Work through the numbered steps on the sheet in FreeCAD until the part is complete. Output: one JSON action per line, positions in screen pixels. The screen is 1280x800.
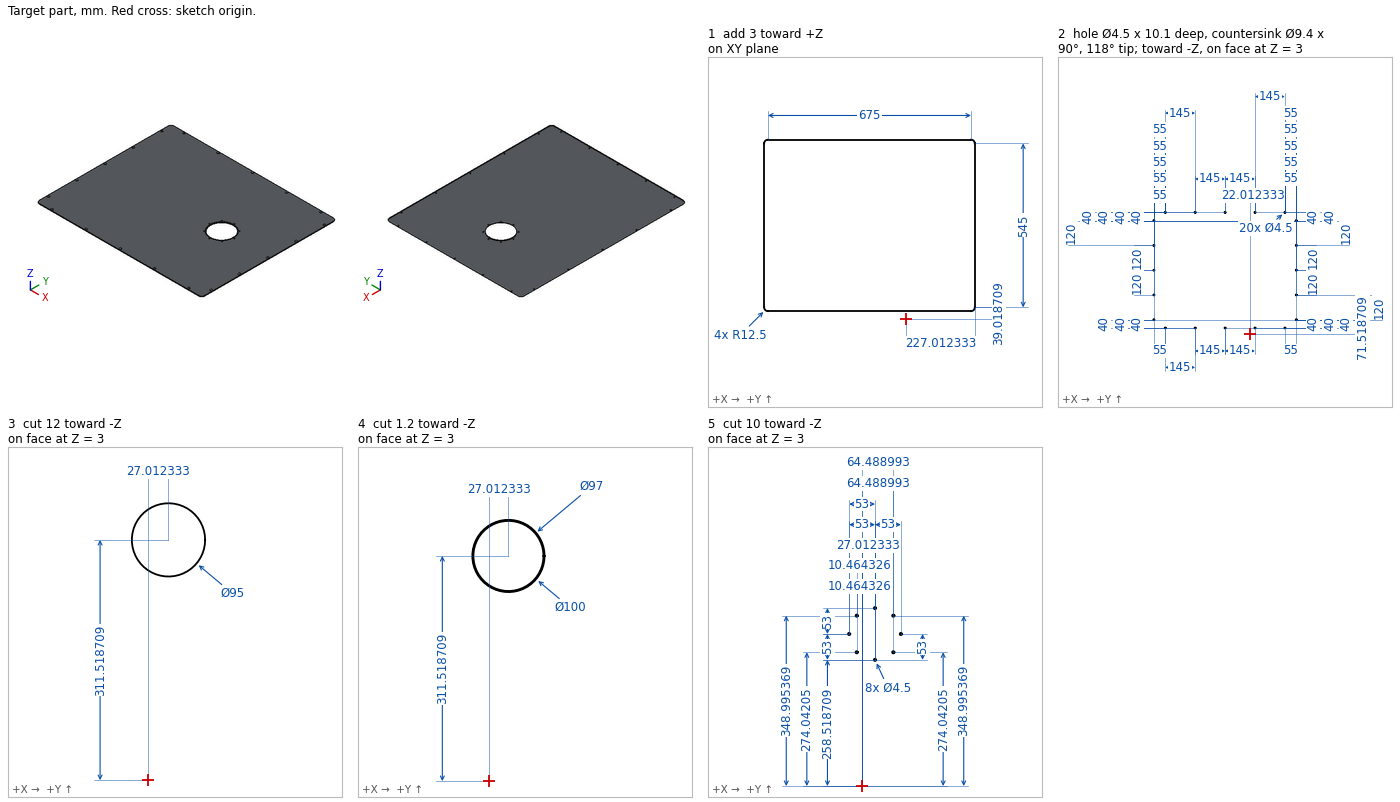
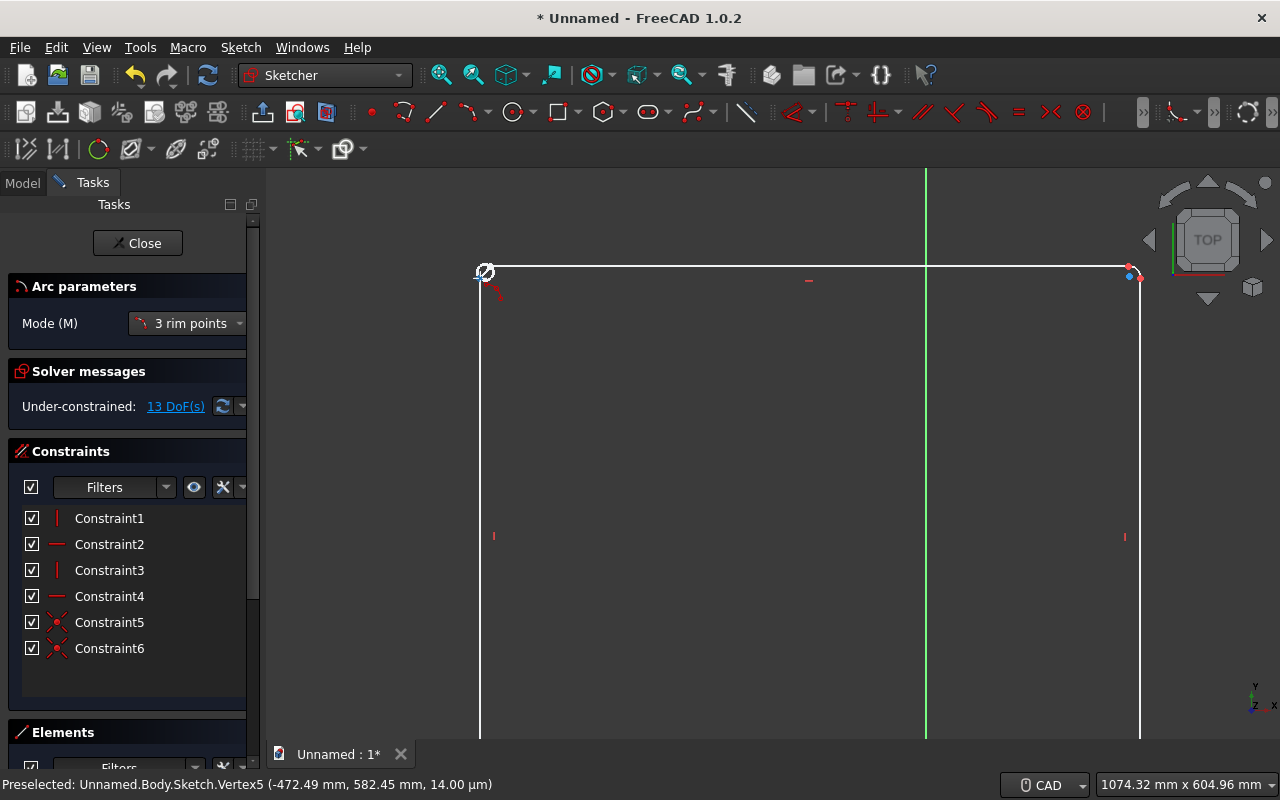
{"action": "scroll", "coordinate": [483, 269], "scroll_direction": "up", "scroll_amount": 8}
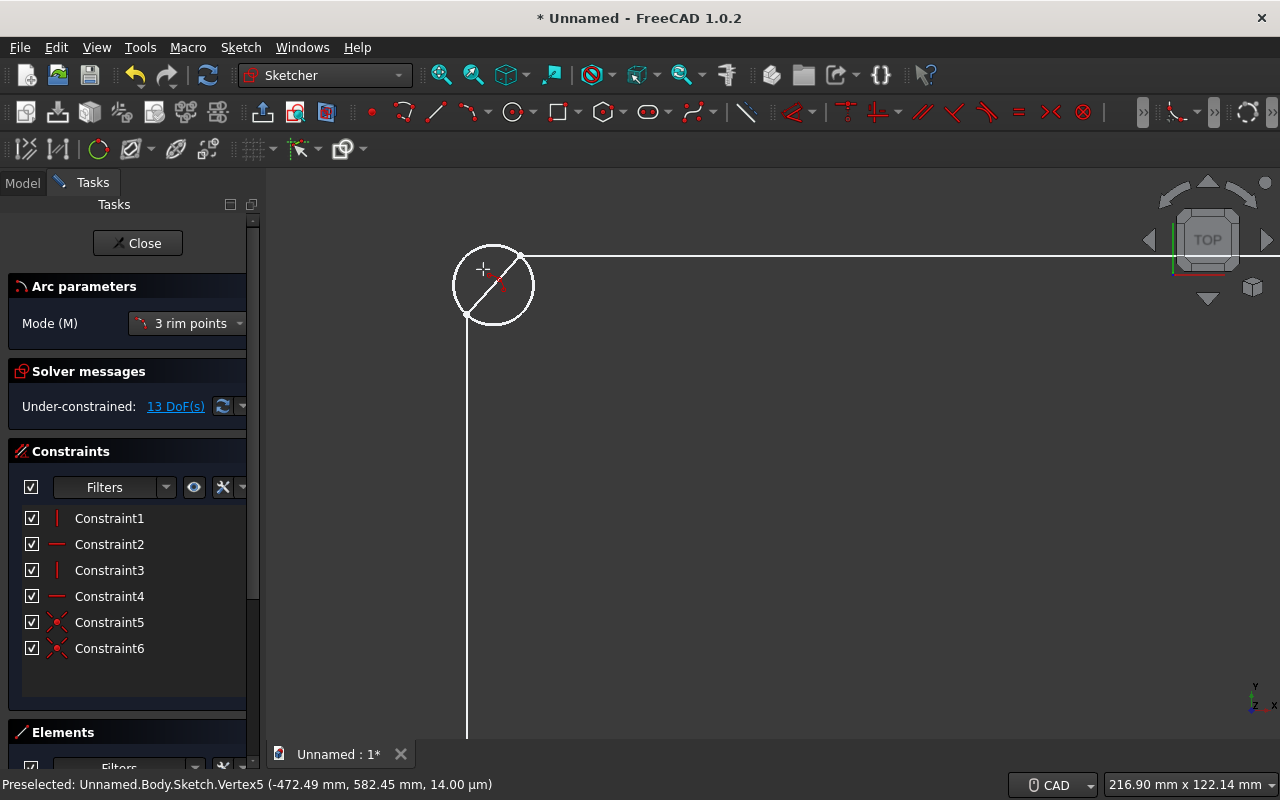
{"action": "left_click", "coordinate": [481, 266]}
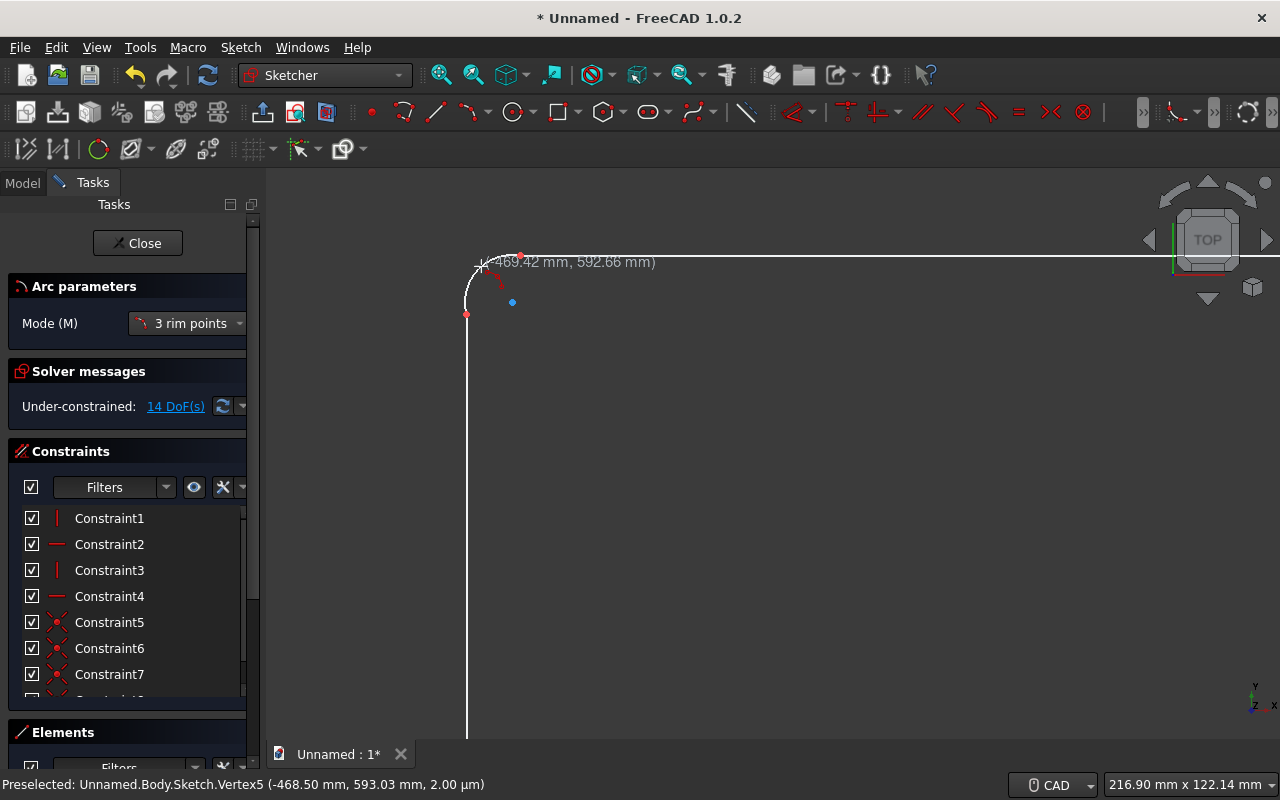
{"action": "scroll", "coordinate": [486, 267], "scroll_direction": "down", "scroll_amount": 10}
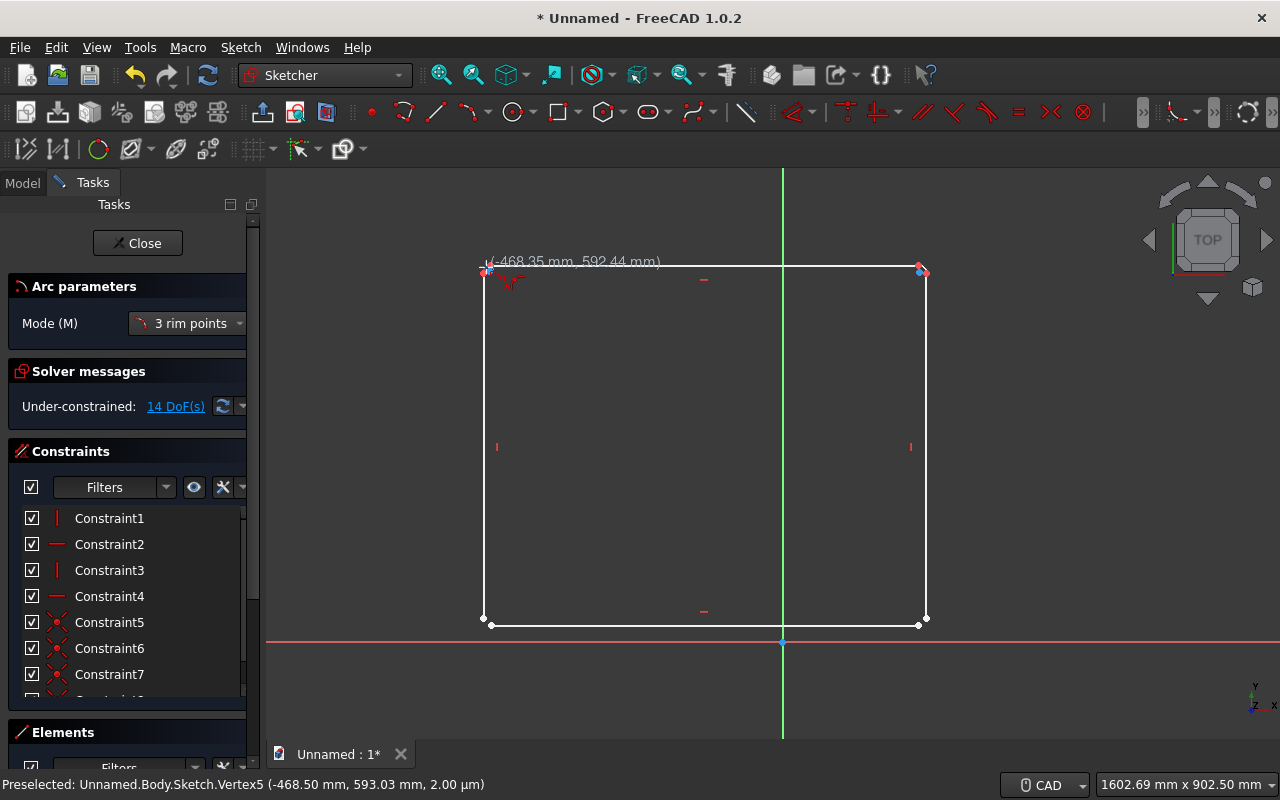
{"action": "scroll", "coordinate": [483, 617], "scroll_direction": "up", "scroll_amount": 2}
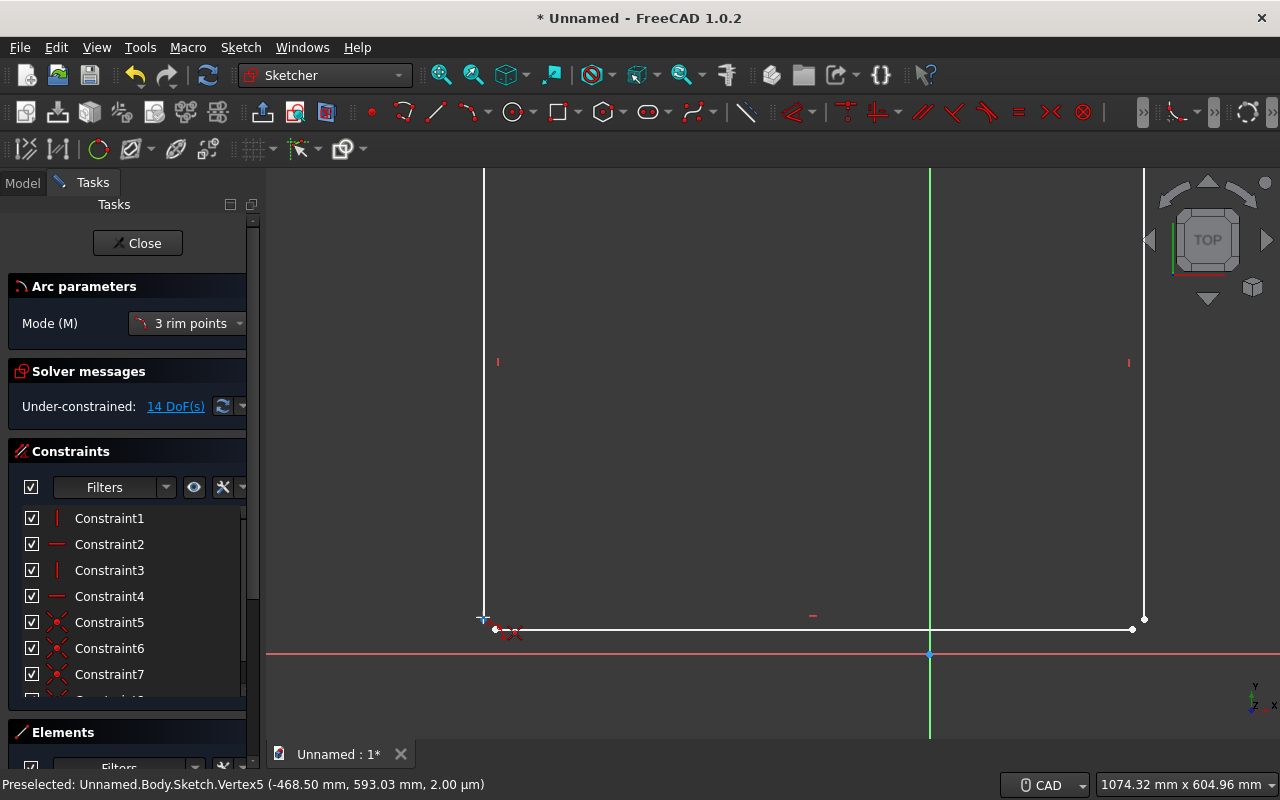
{"action": "left_click", "coordinate": [484, 619]}
{"action": "left_click", "coordinate": [495, 630]}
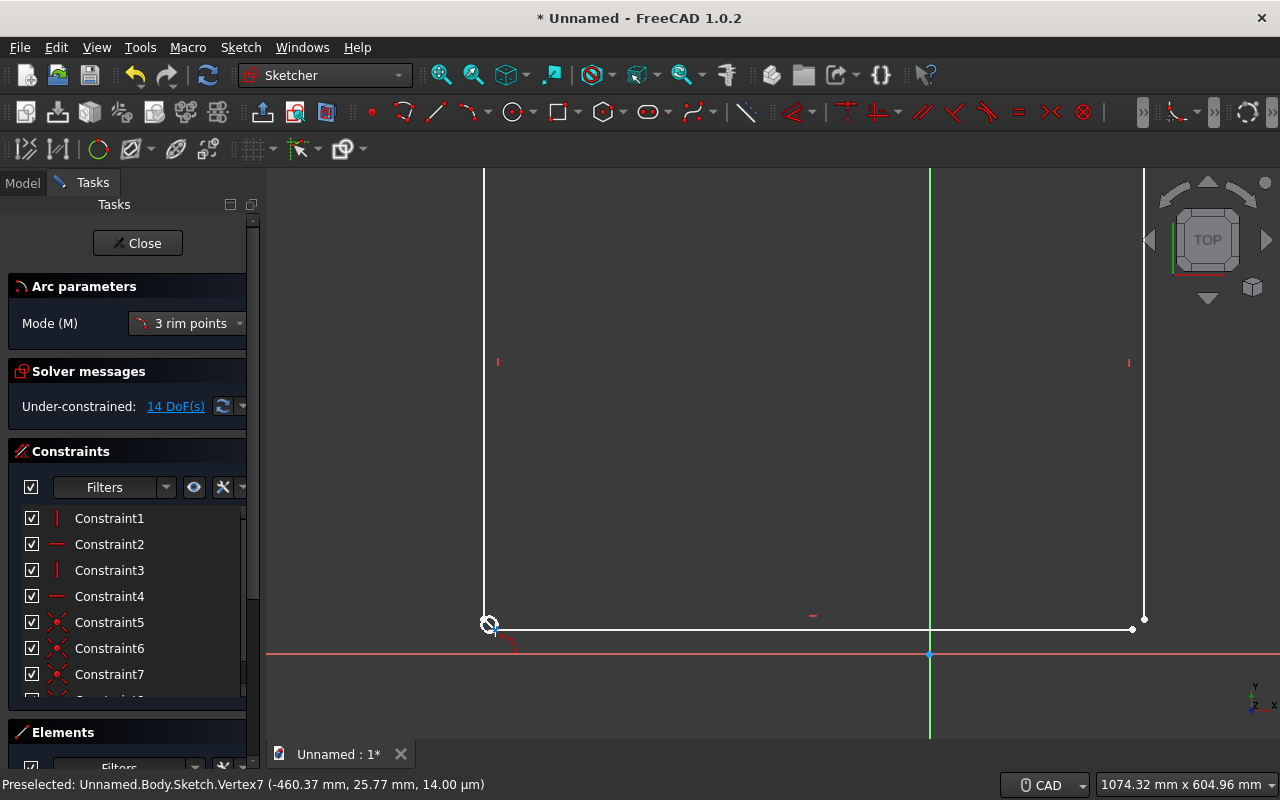
{"action": "scroll", "coordinate": [487, 626], "scroll_direction": "up", "scroll_amount": 8}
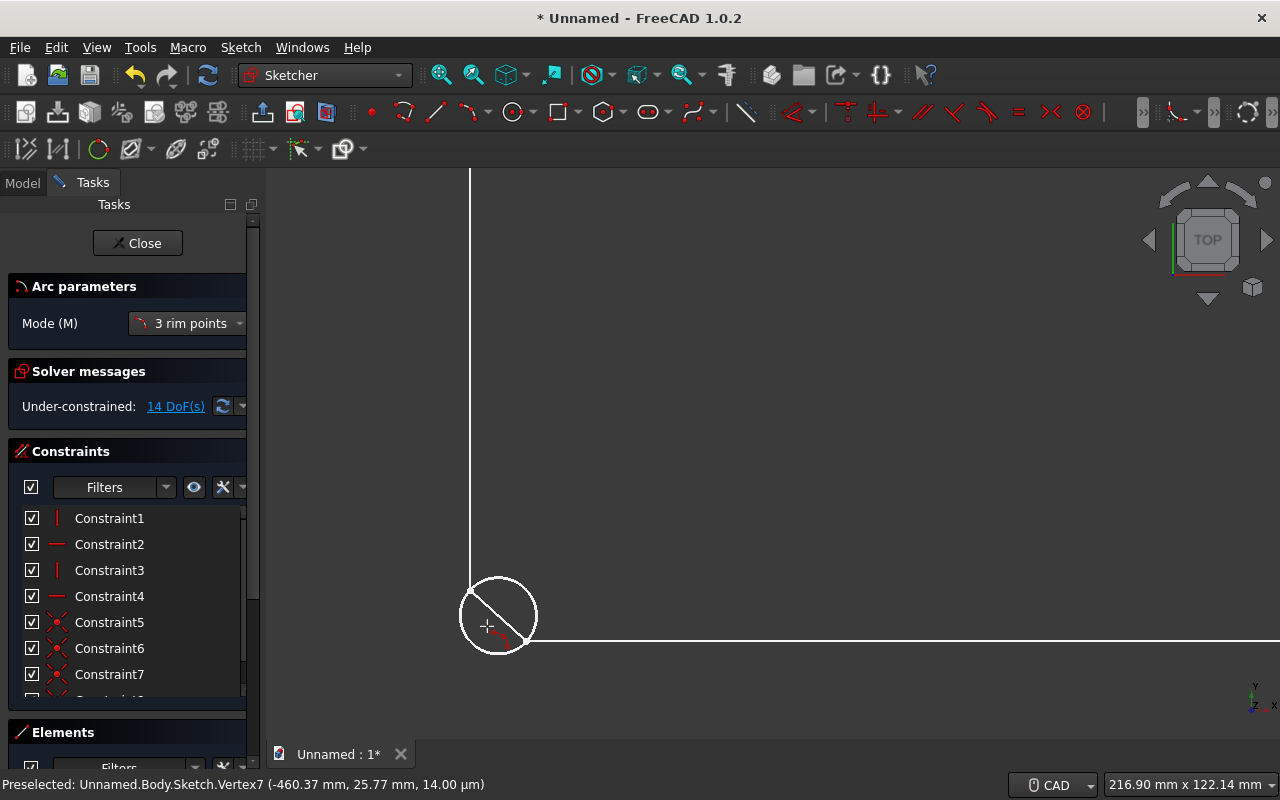
{"action": "left_click", "coordinate": [485, 621]}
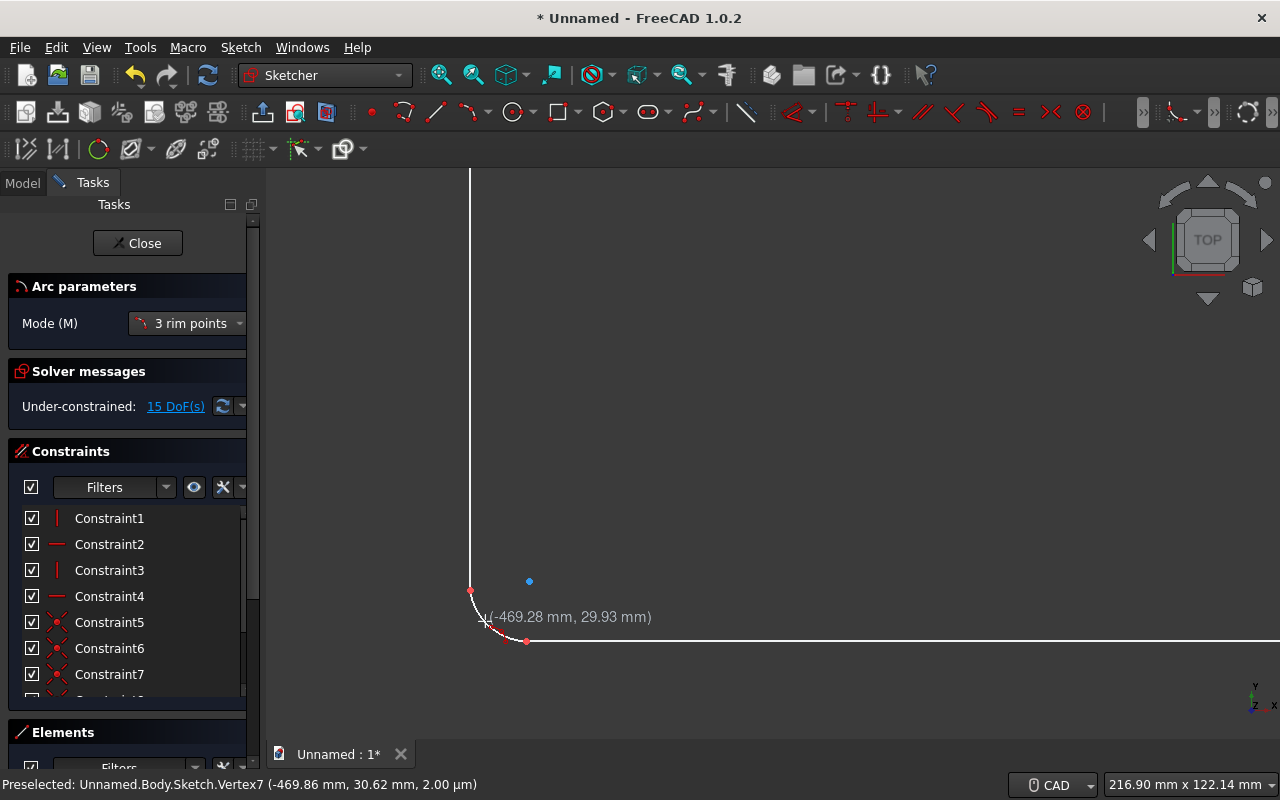
{"action": "scroll", "coordinate": [485, 623], "scroll_direction": "down", "scroll_amount": 10}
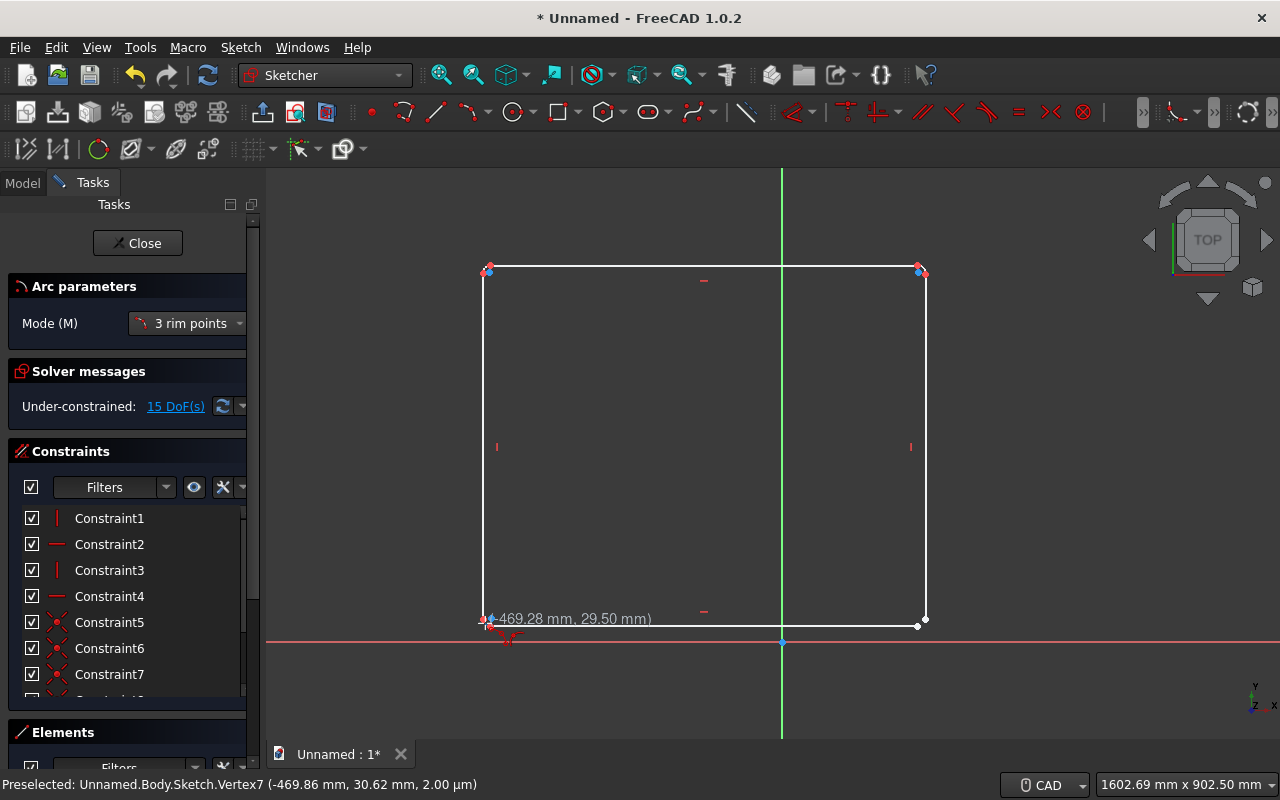
{"action": "scroll", "coordinate": [918, 626], "scroll_direction": "up", "scroll_amount": 2}